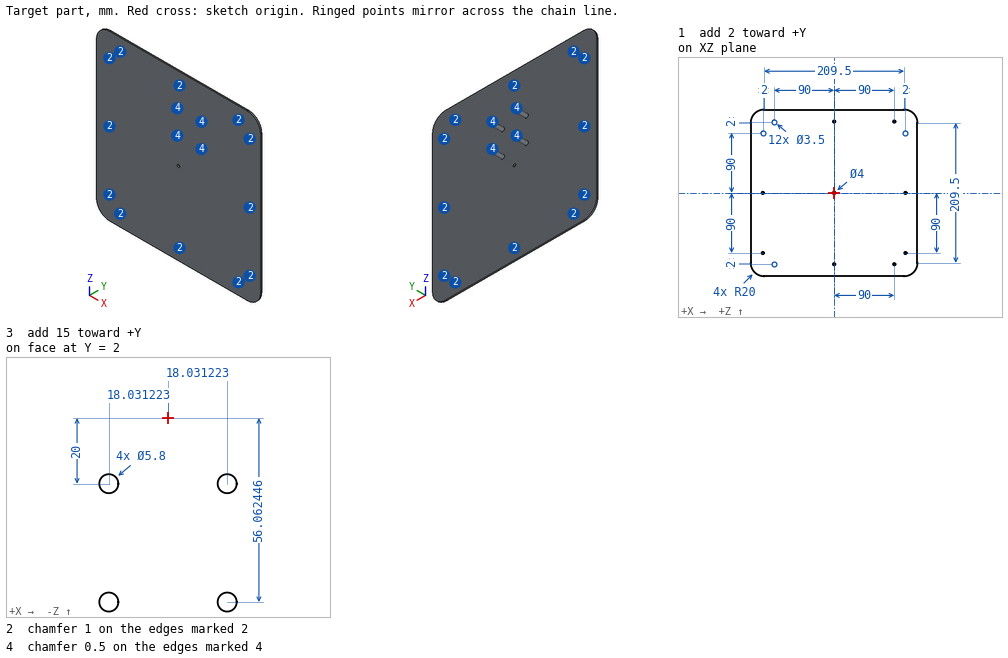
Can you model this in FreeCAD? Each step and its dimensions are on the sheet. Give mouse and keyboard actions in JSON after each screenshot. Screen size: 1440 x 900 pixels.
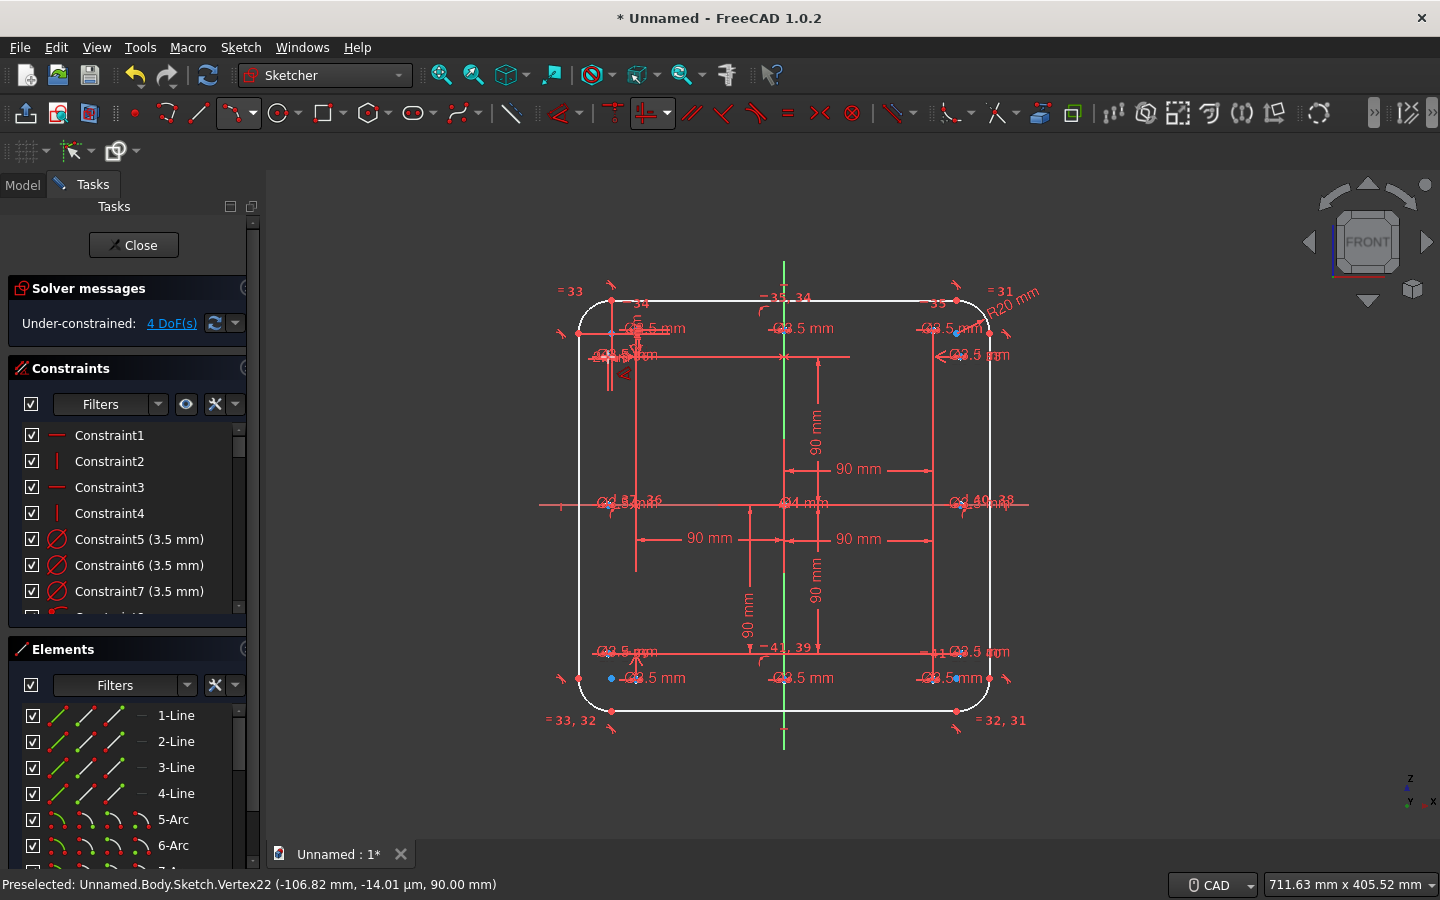
{"action": "scroll", "coordinate": [957, 301], "scroll_direction": "up", "scroll_amount": 13}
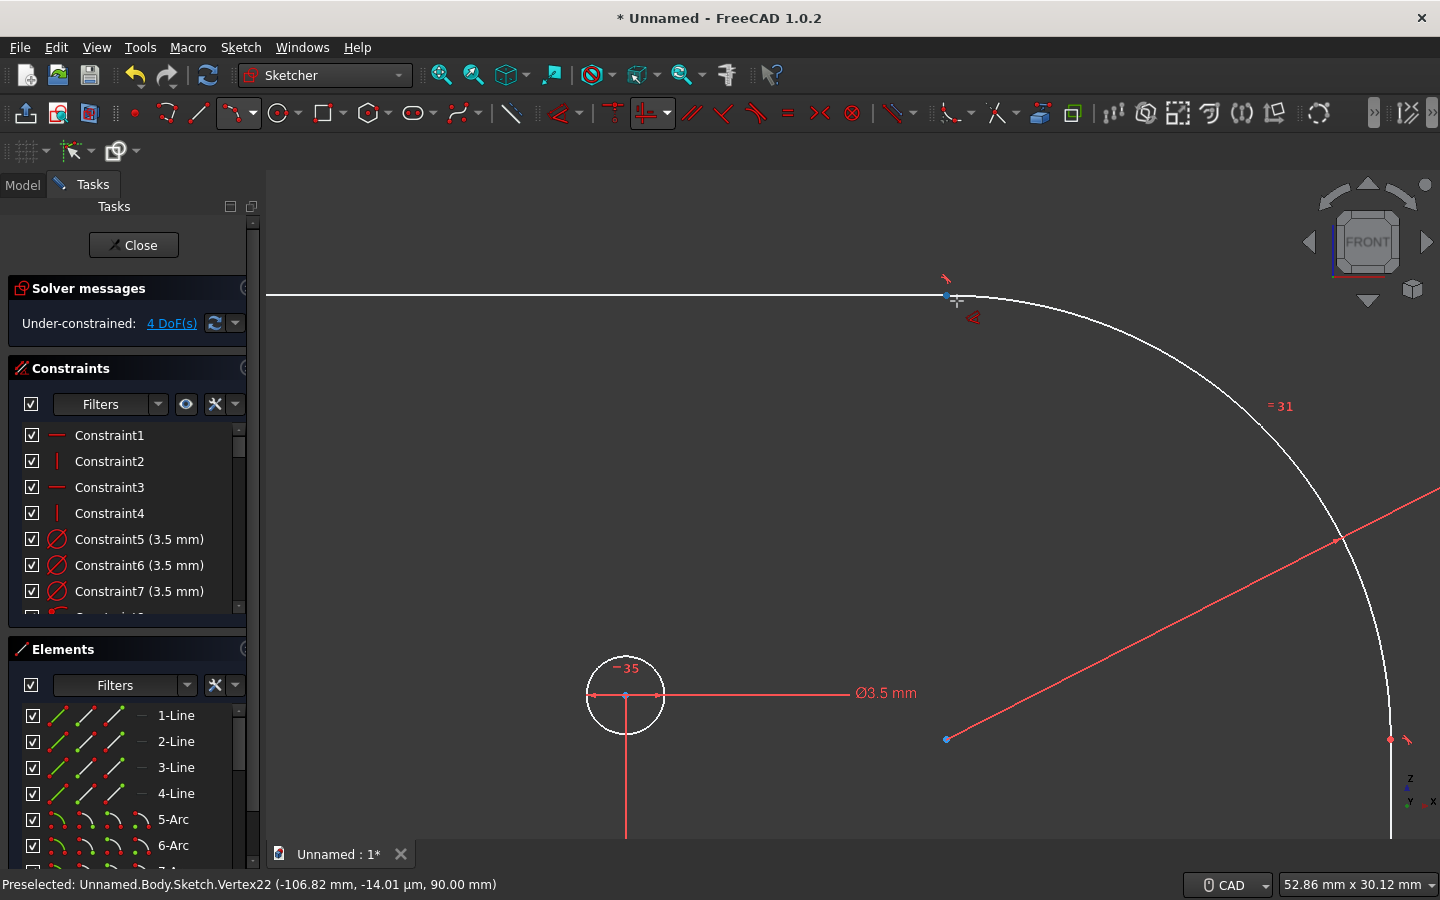
{"action": "left_click", "coordinate": [947, 295]}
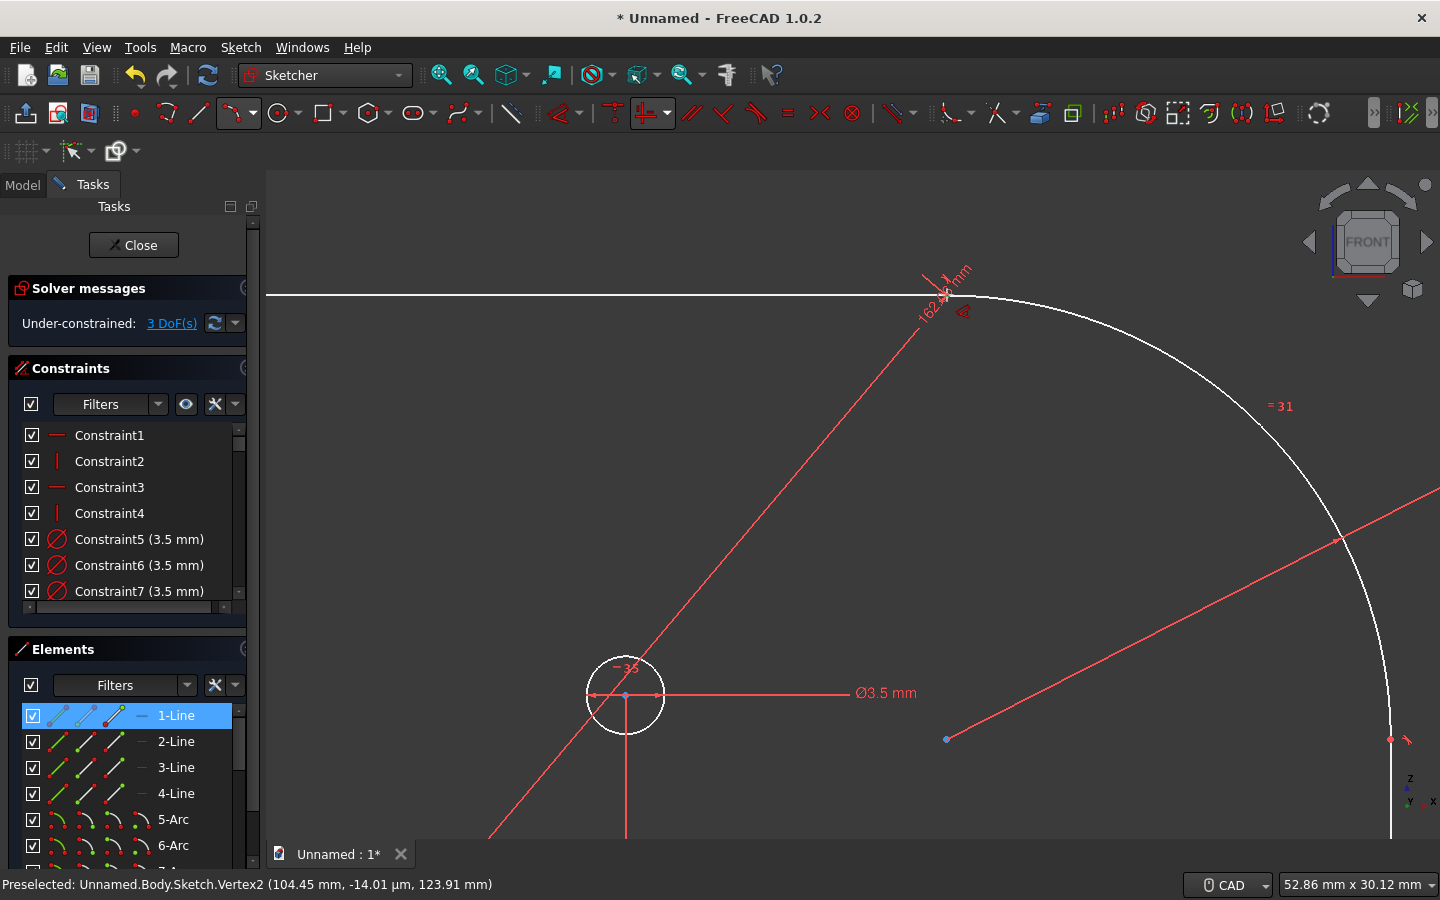
{"action": "scroll", "coordinate": [958, 300], "scroll_direction": "down", "scroll_amount": 13}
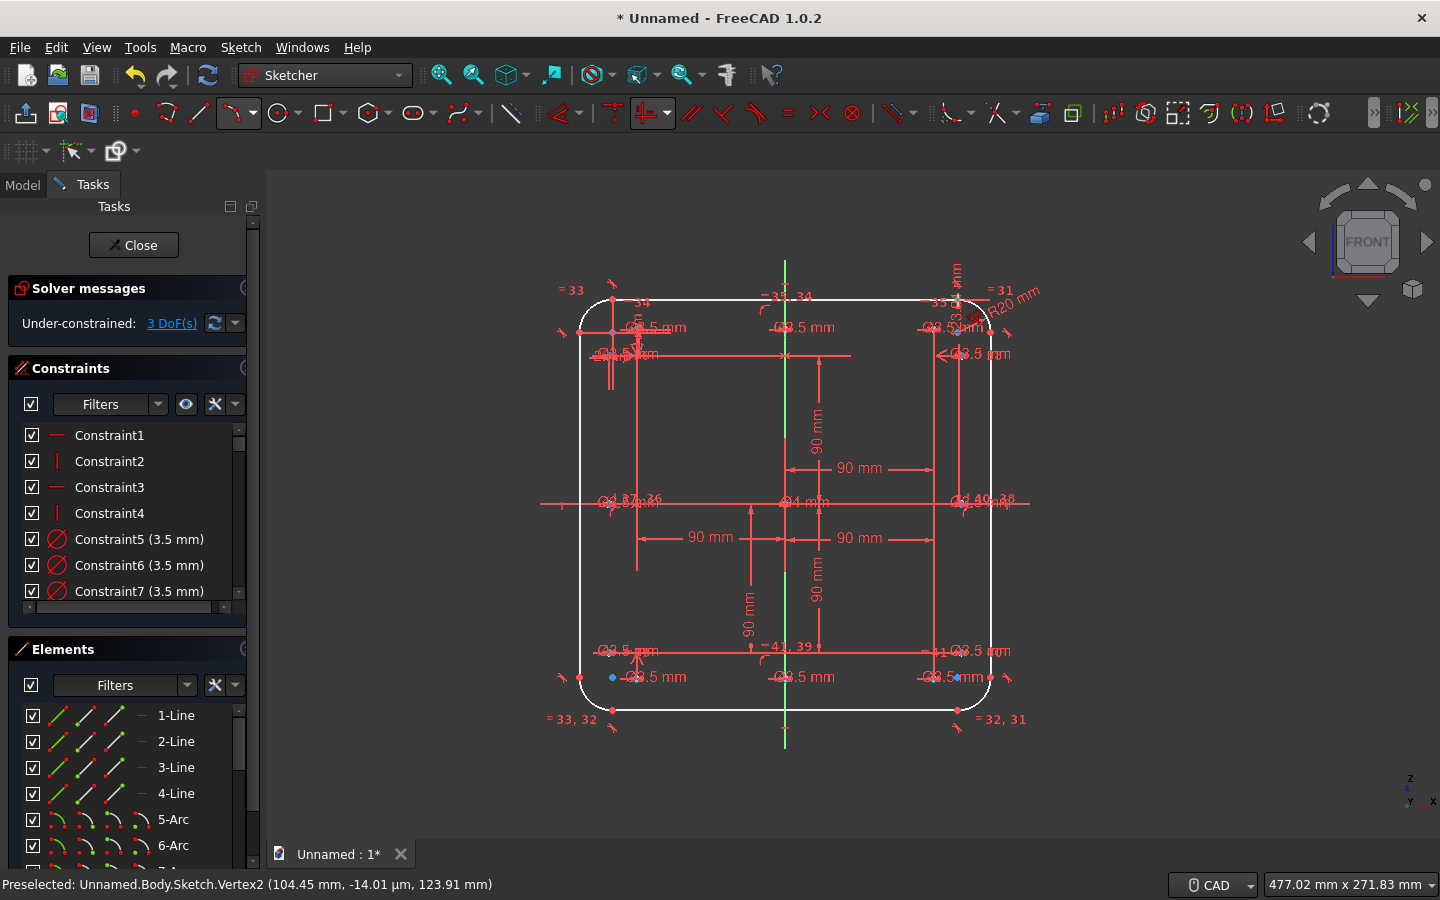
{"action": "scroll", "coordinate": [962, 356], "scroll_direction": "up", "scroll_amount": 13}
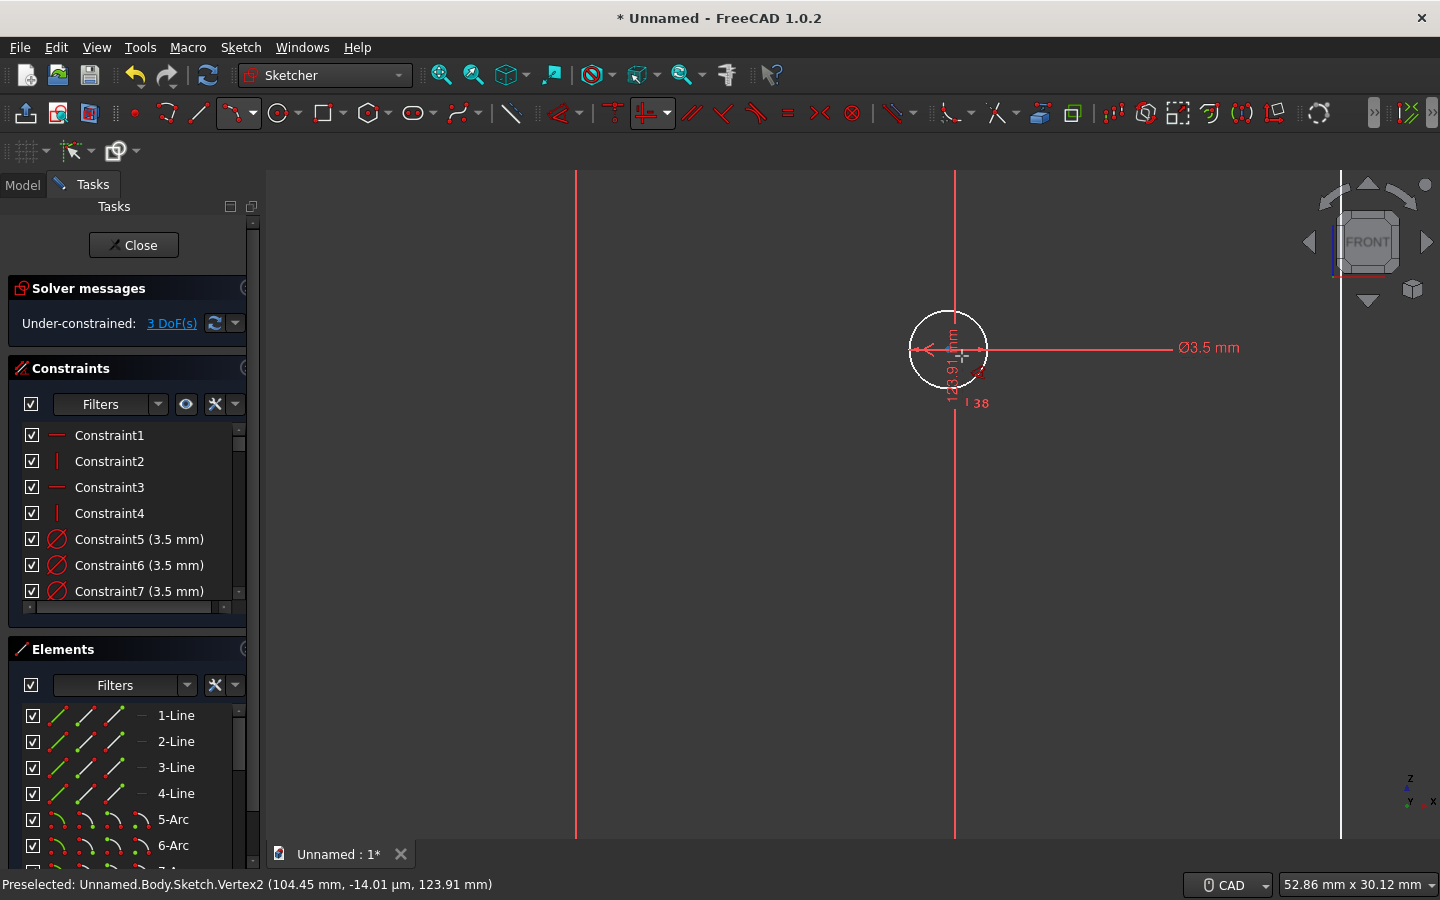
{"action": "left_click", "coordinate": [948, 350]}
{"action": "left_click", "coordinate": [904, 384]}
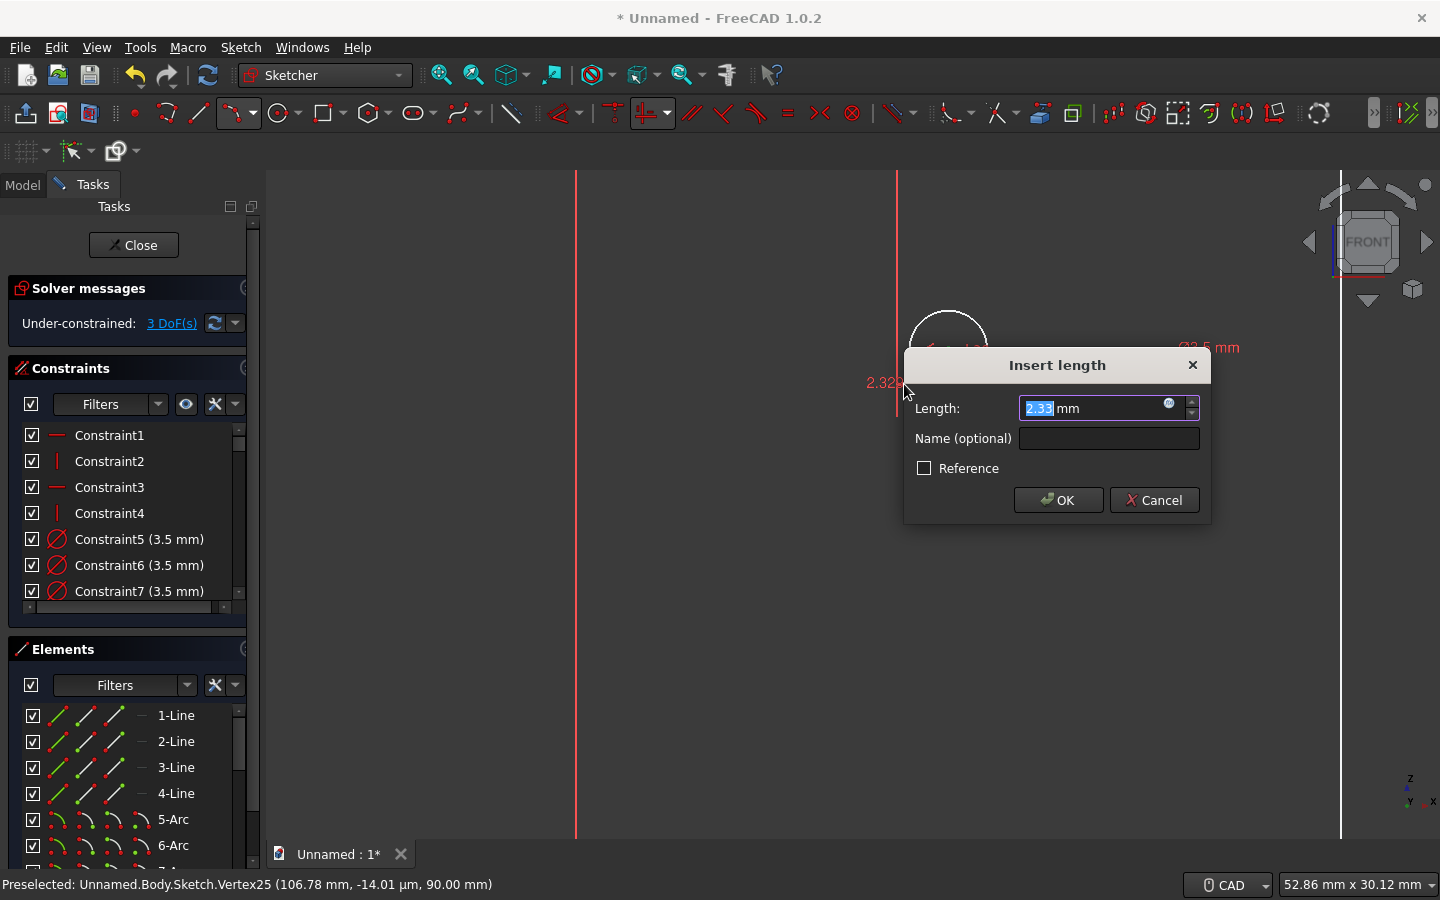
{"action": "type", "text": "2"}
{"action": "key", "text": "Return"}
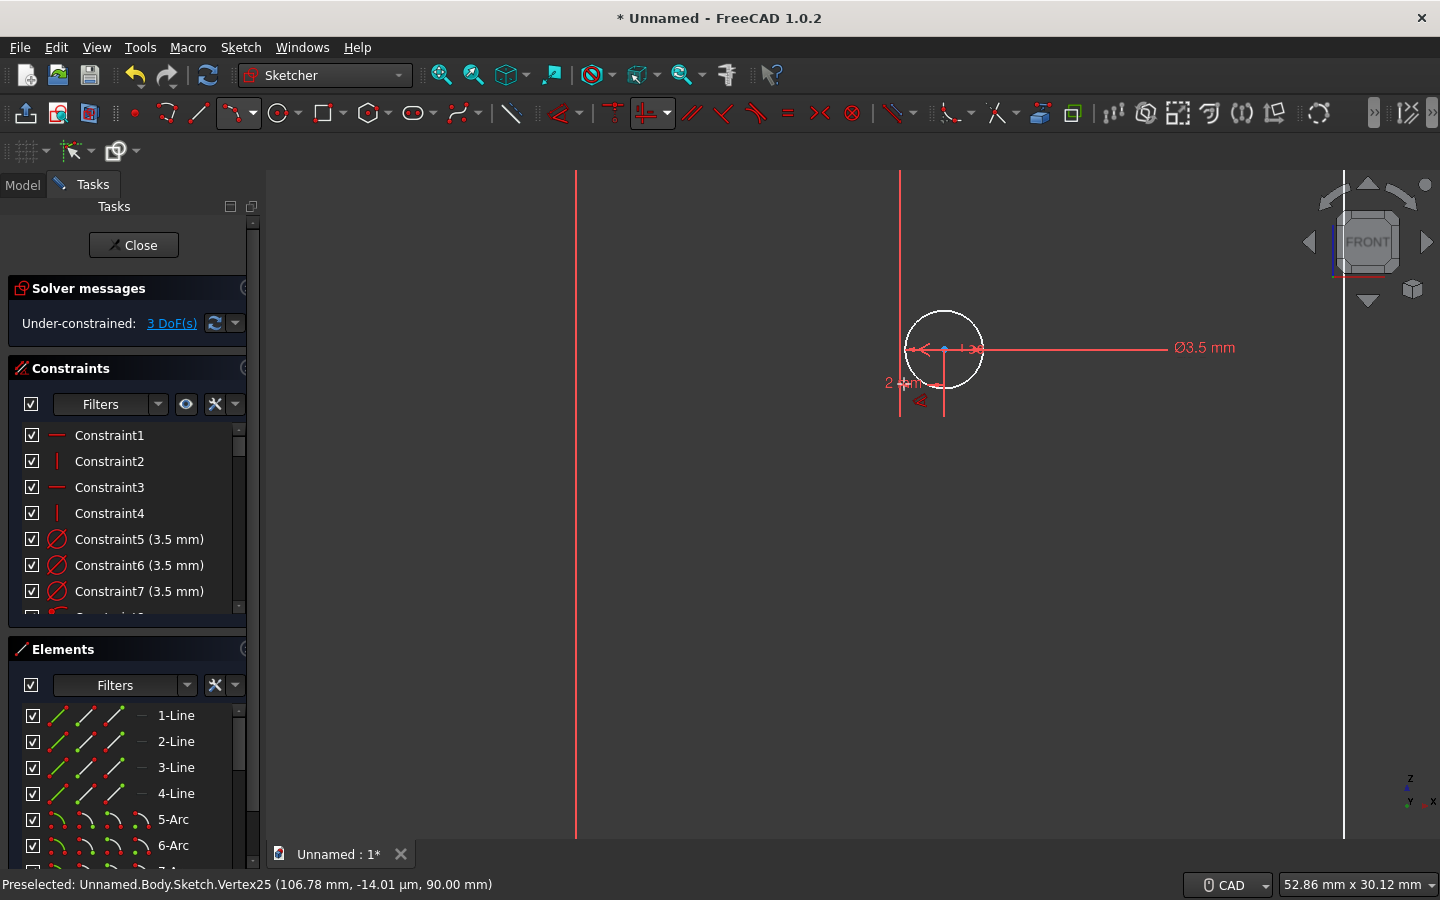
{"action": "scroll", "coordinate": [962, 357], "scroll_direction": "down", "scroll_amount": 13}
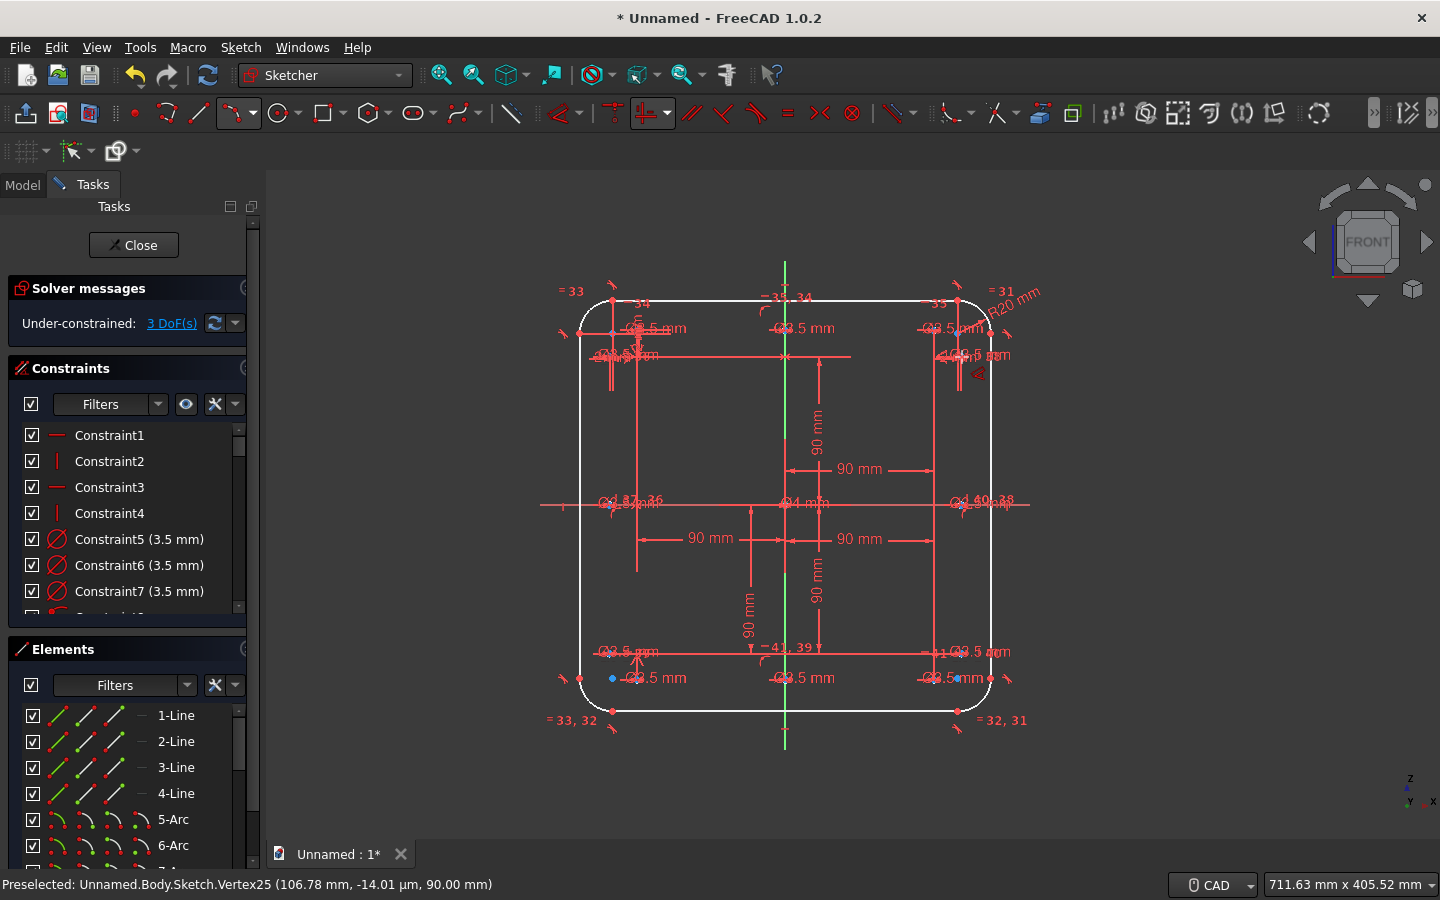
{"action": "scroll", "coordinate": [580, 678], "scroll_direction": "up", "scroll_amount": 13}